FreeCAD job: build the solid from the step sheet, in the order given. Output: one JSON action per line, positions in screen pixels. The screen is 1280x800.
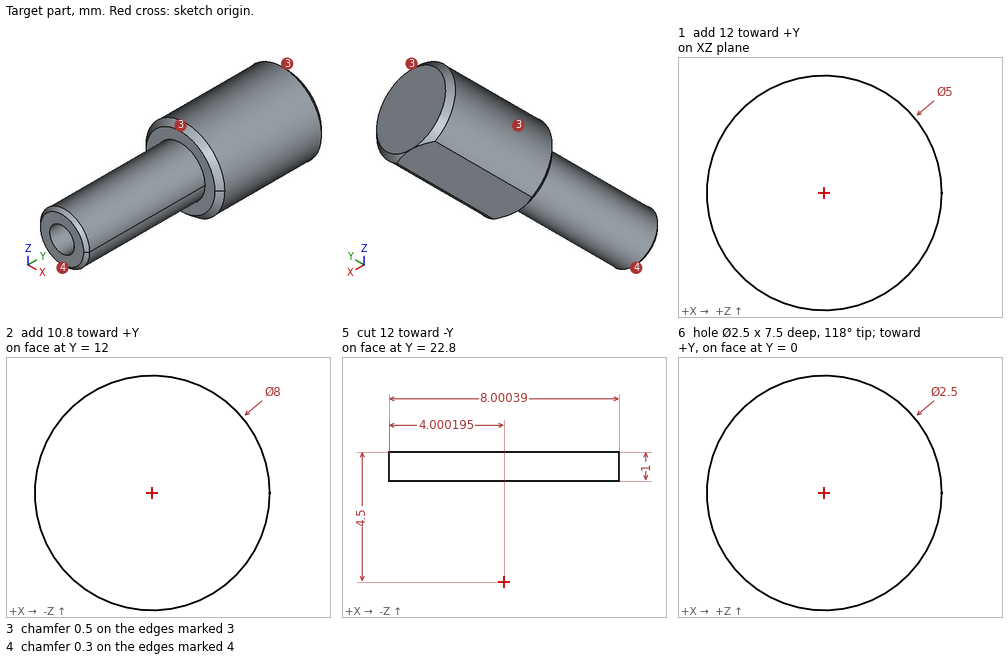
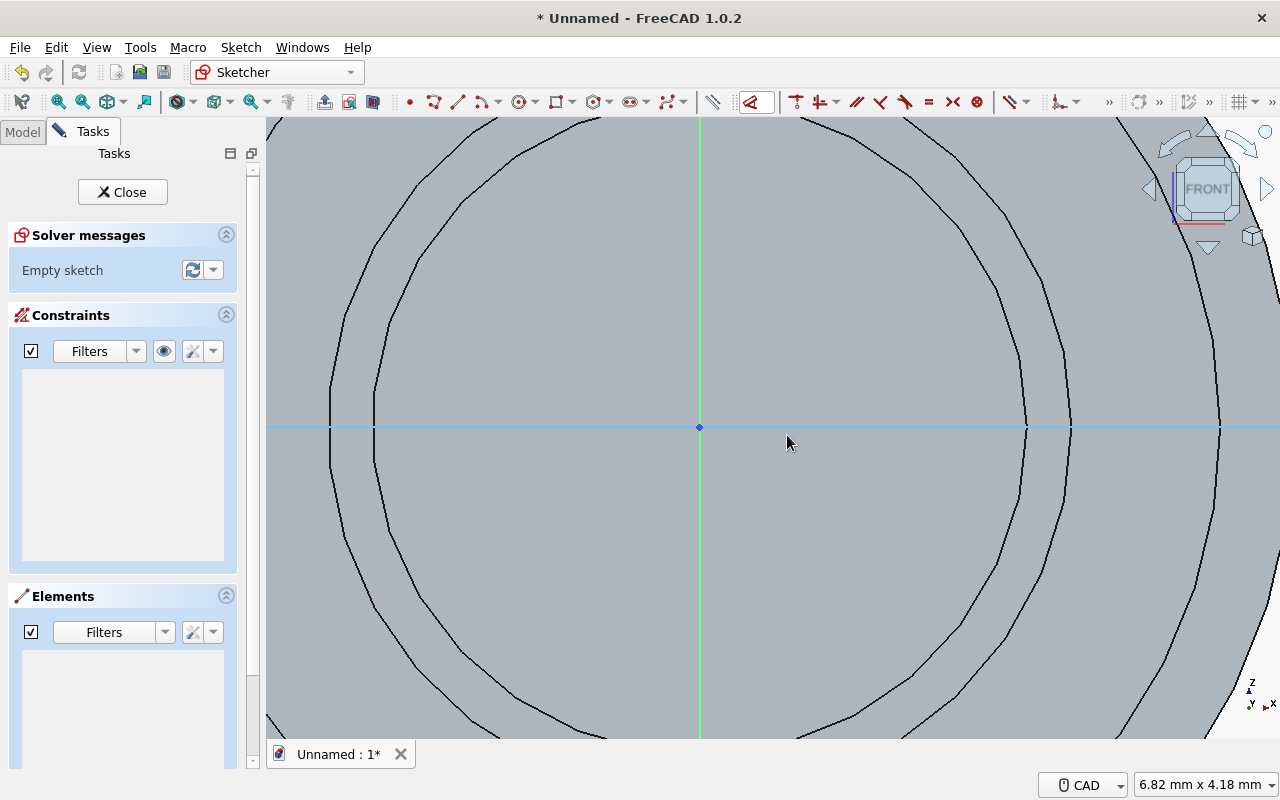
{"action": "left_click", "coordinate": [520, 102]}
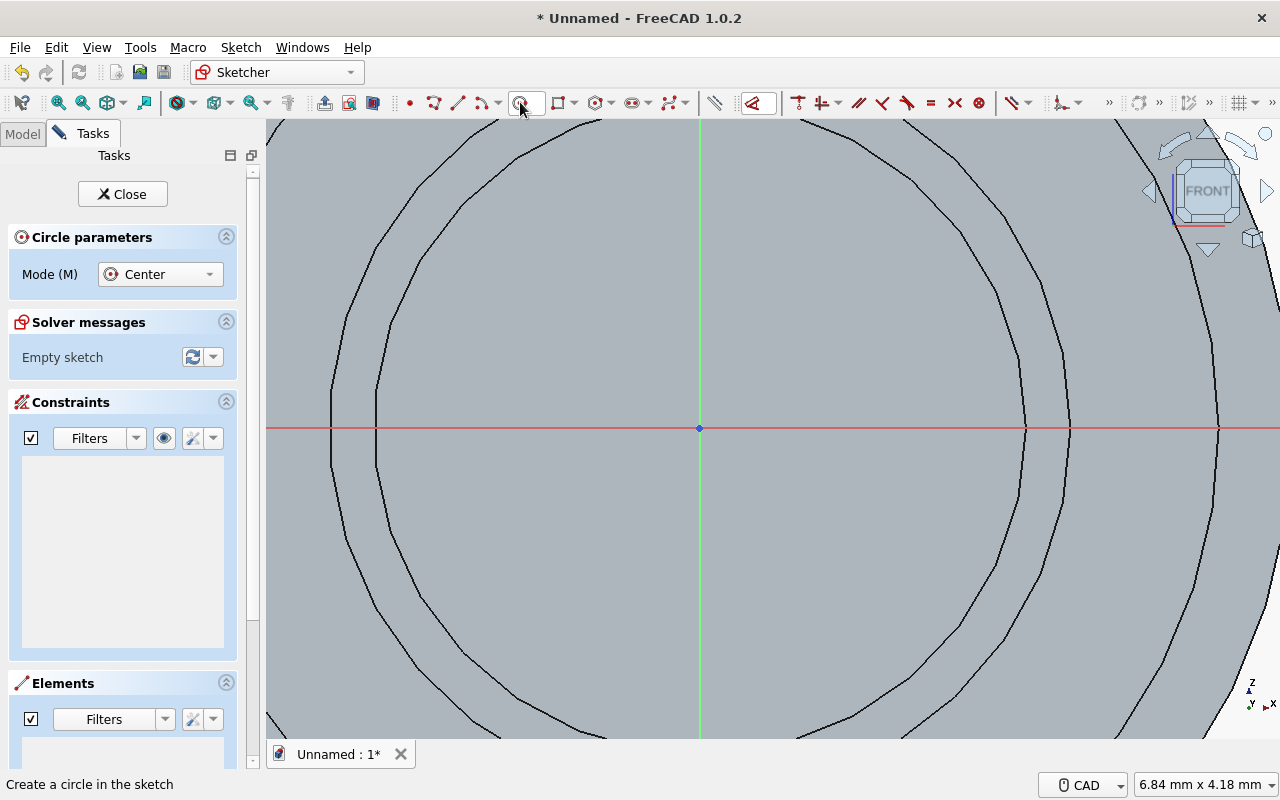
{"action": "left_click", "coordinate": [700, 428]}
{"action": "mouse_move", "coordinate": [831, 297]}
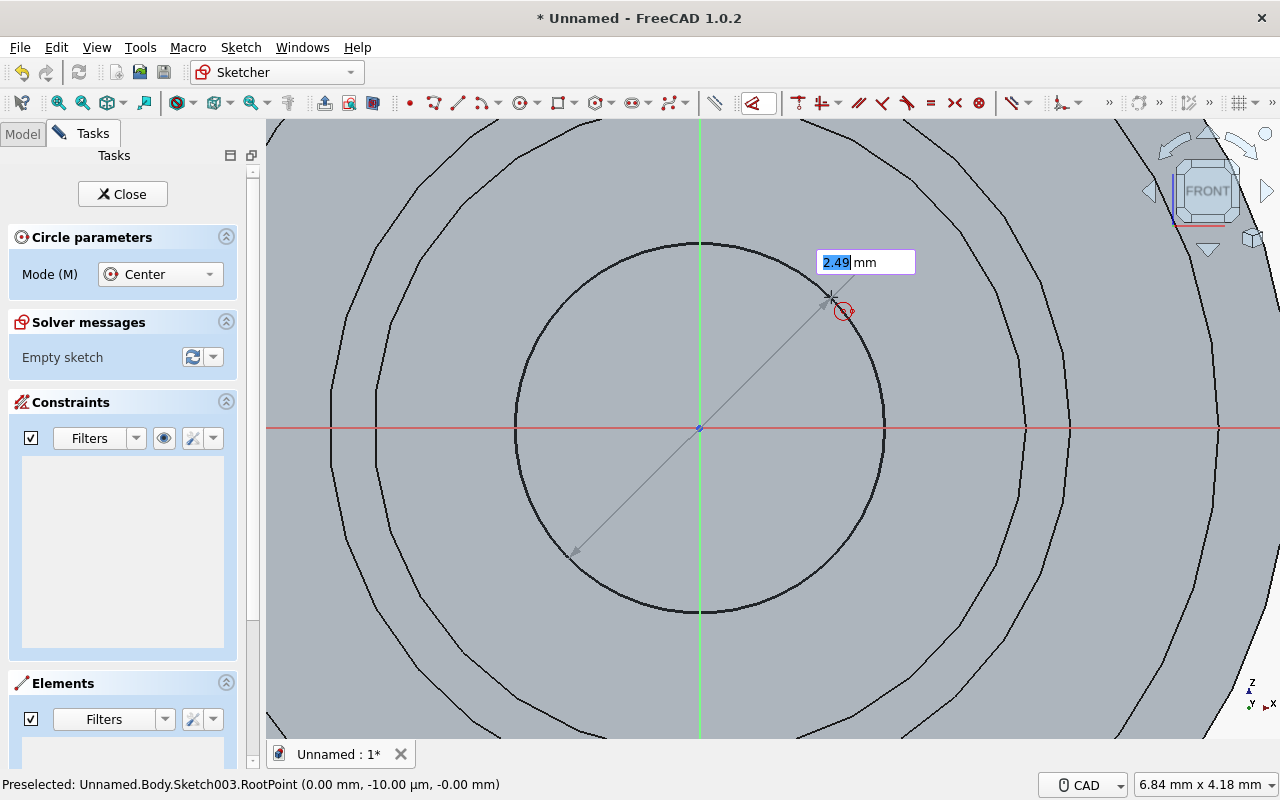
{"action": "type", "text": "2.5"}
{"action": "key", "text": "Return"}
{"action": "key", "text": "Escape"}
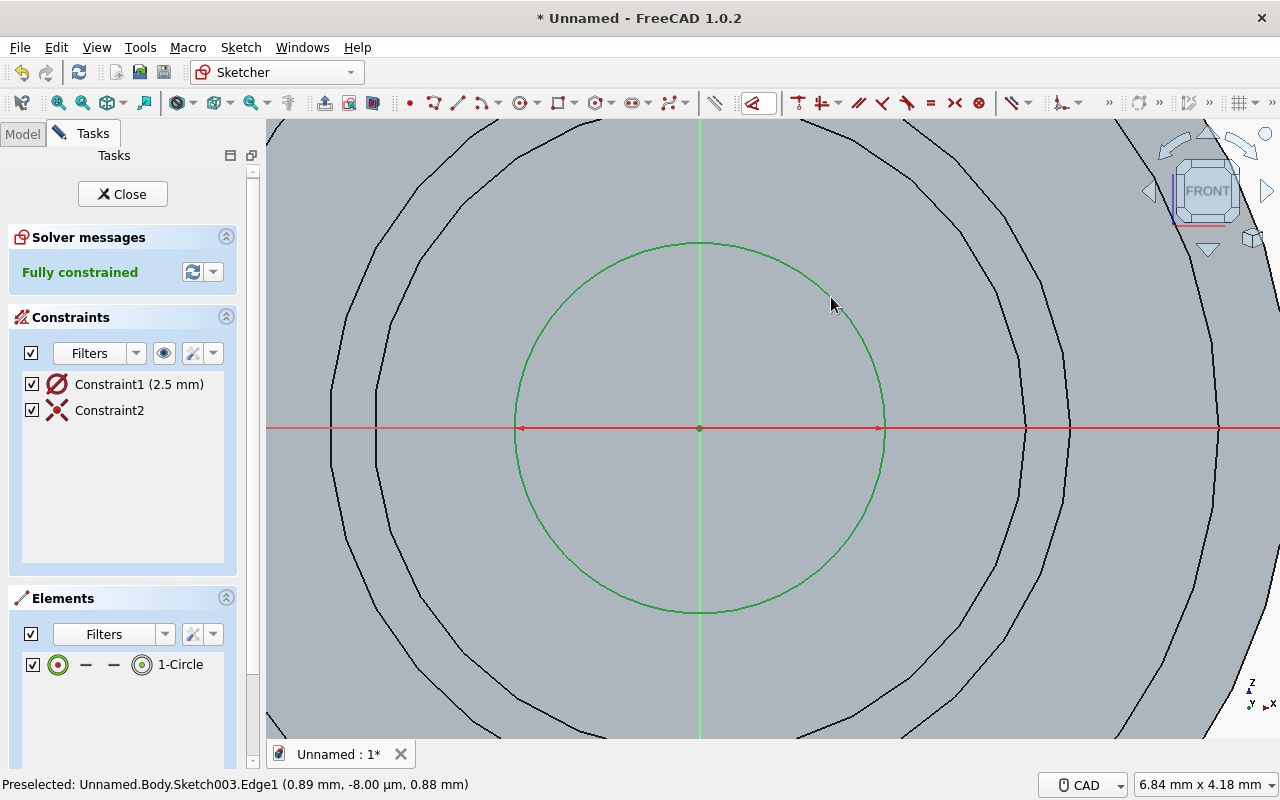
{"action": "left_click", "coordinate": [123, 194]}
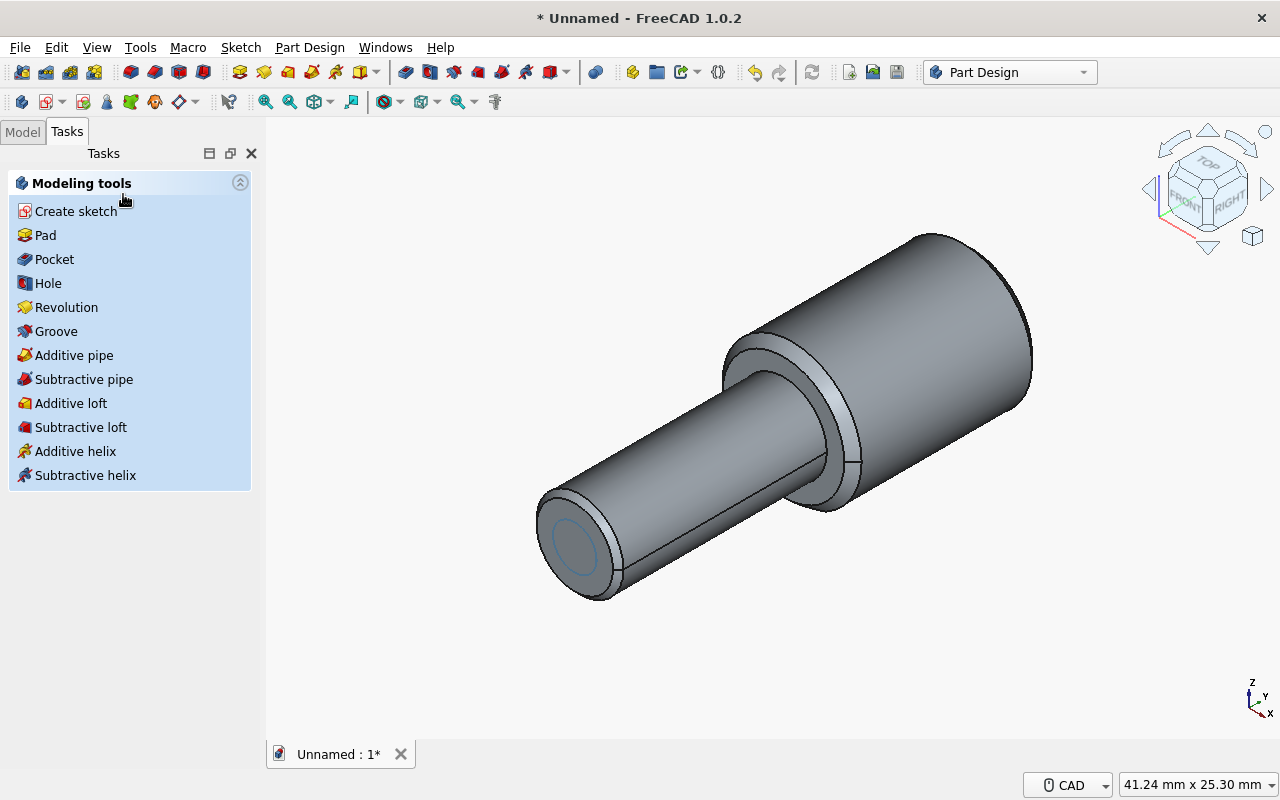
{"action": "left_click", "coordinate": [430, 72]}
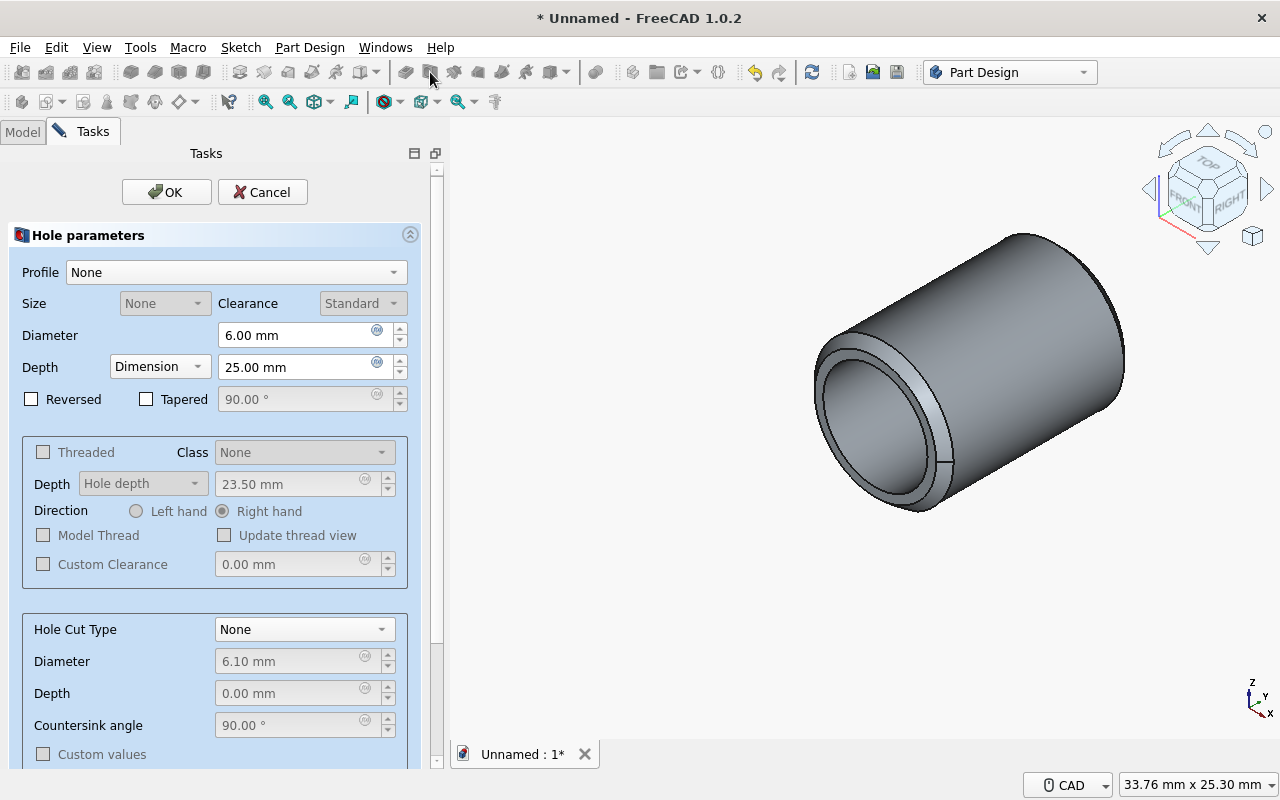
{"action": "triple_click", "coordinate": [305, 335]}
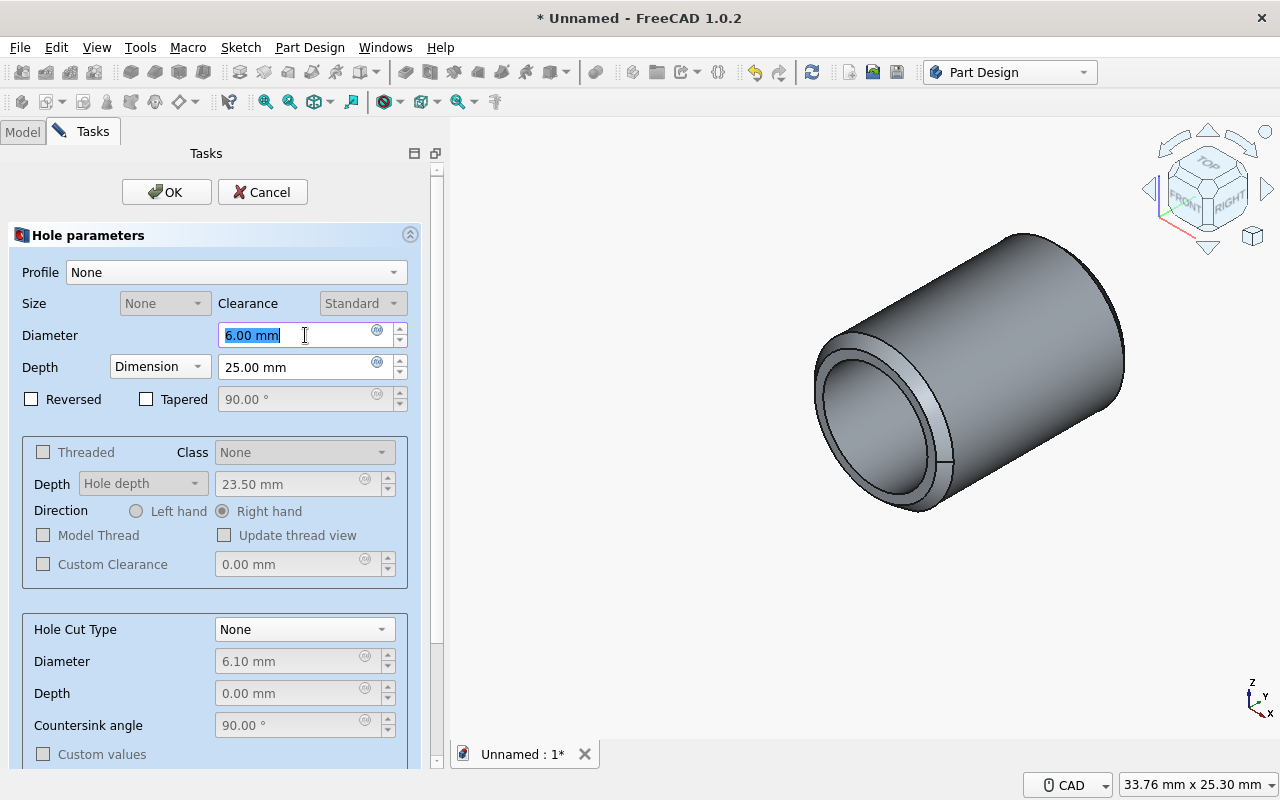
{"action": "type", "text": "2.5"}
{"action": "key", "text": "Tab"}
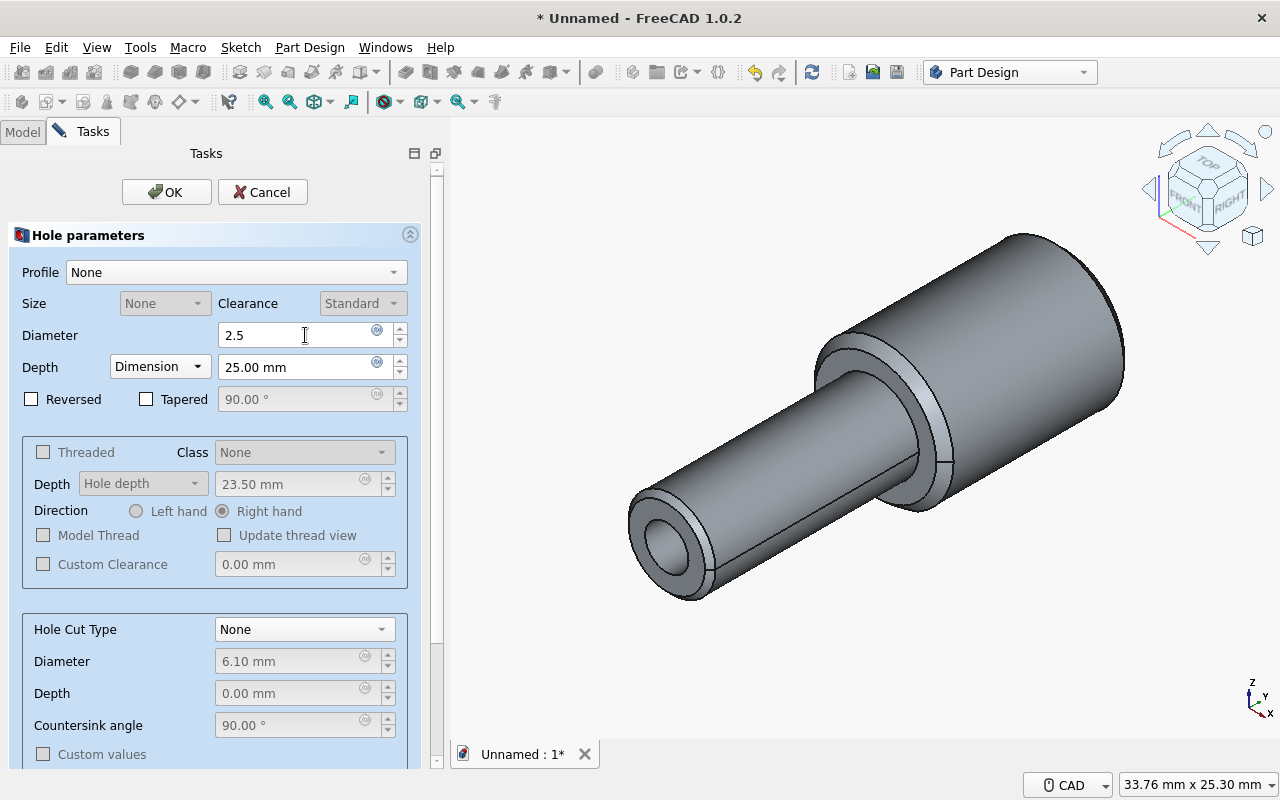
{"action": "triple_click", "coordinate": [305, 367]}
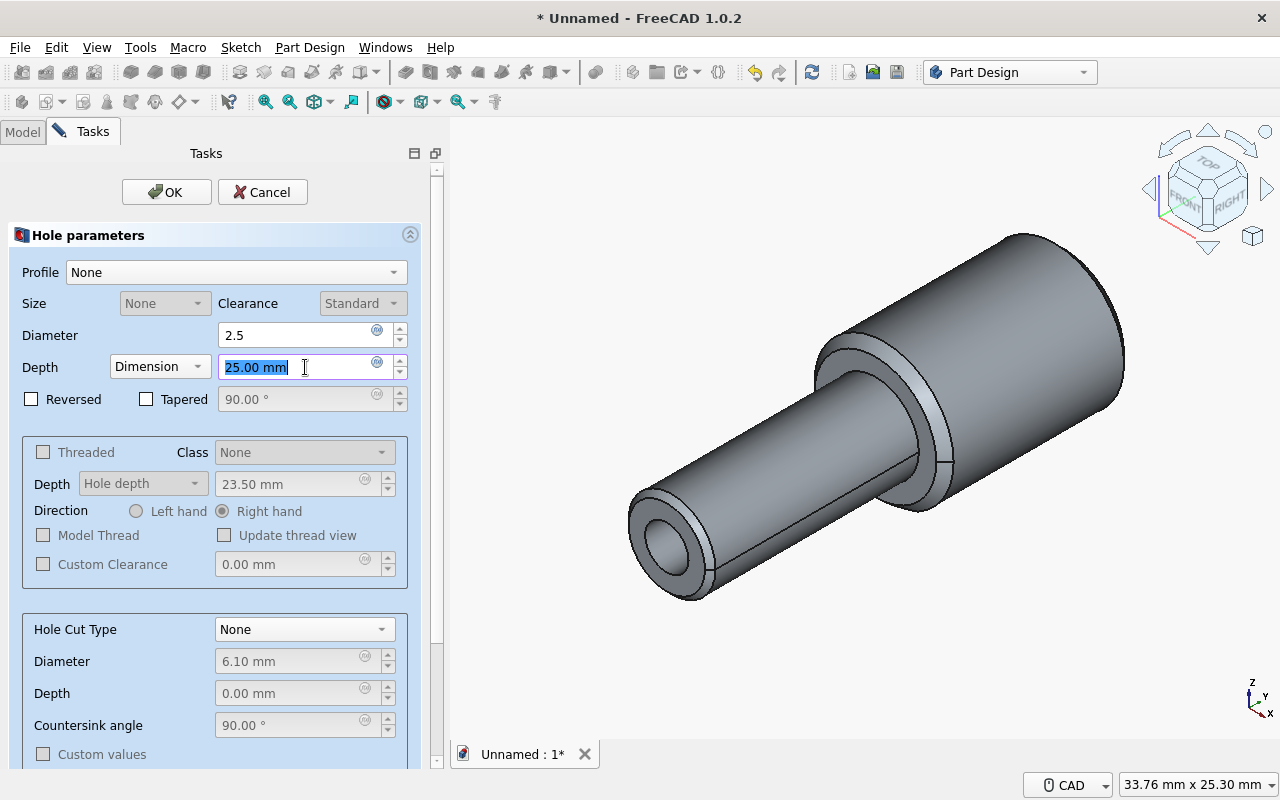
{"action": "type", "text": "7.5"}
{"action": "key", "text": "Tab"}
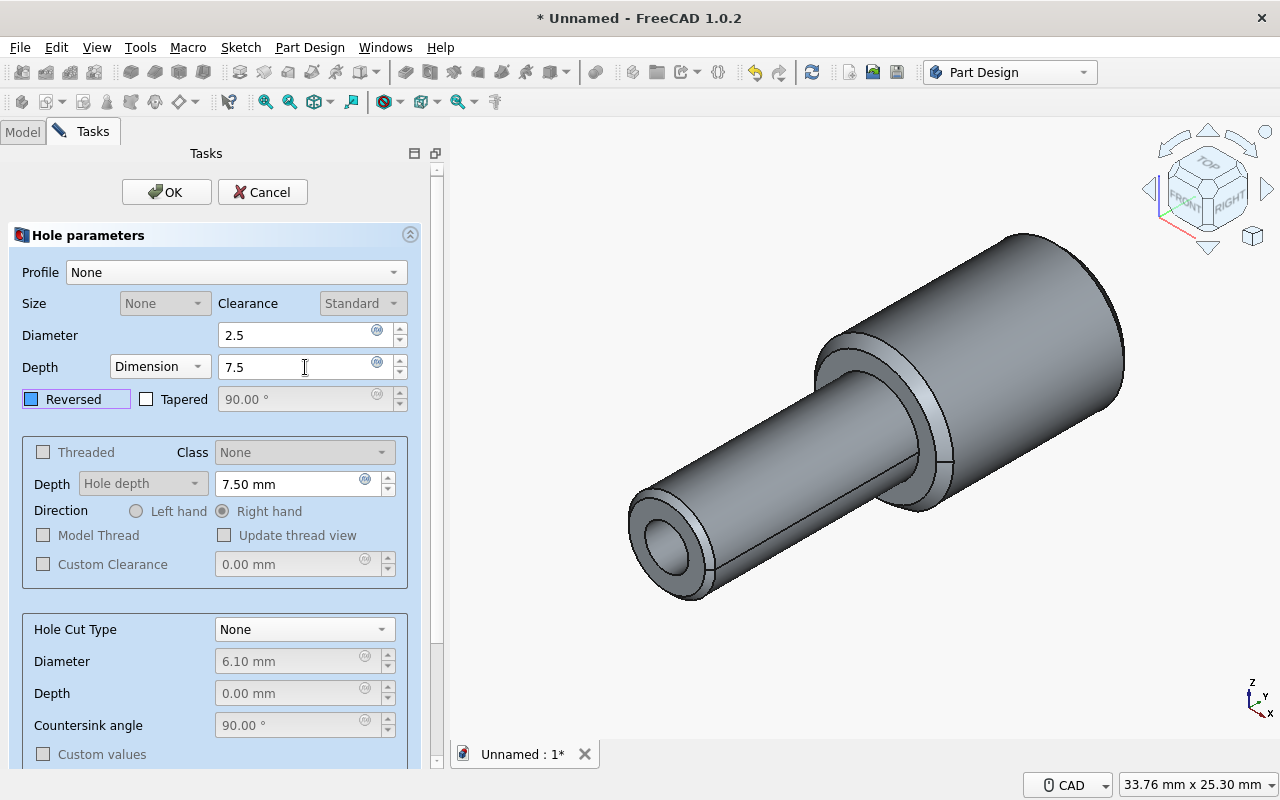
{"action": "left_click", "coordinate": [167, 192]}